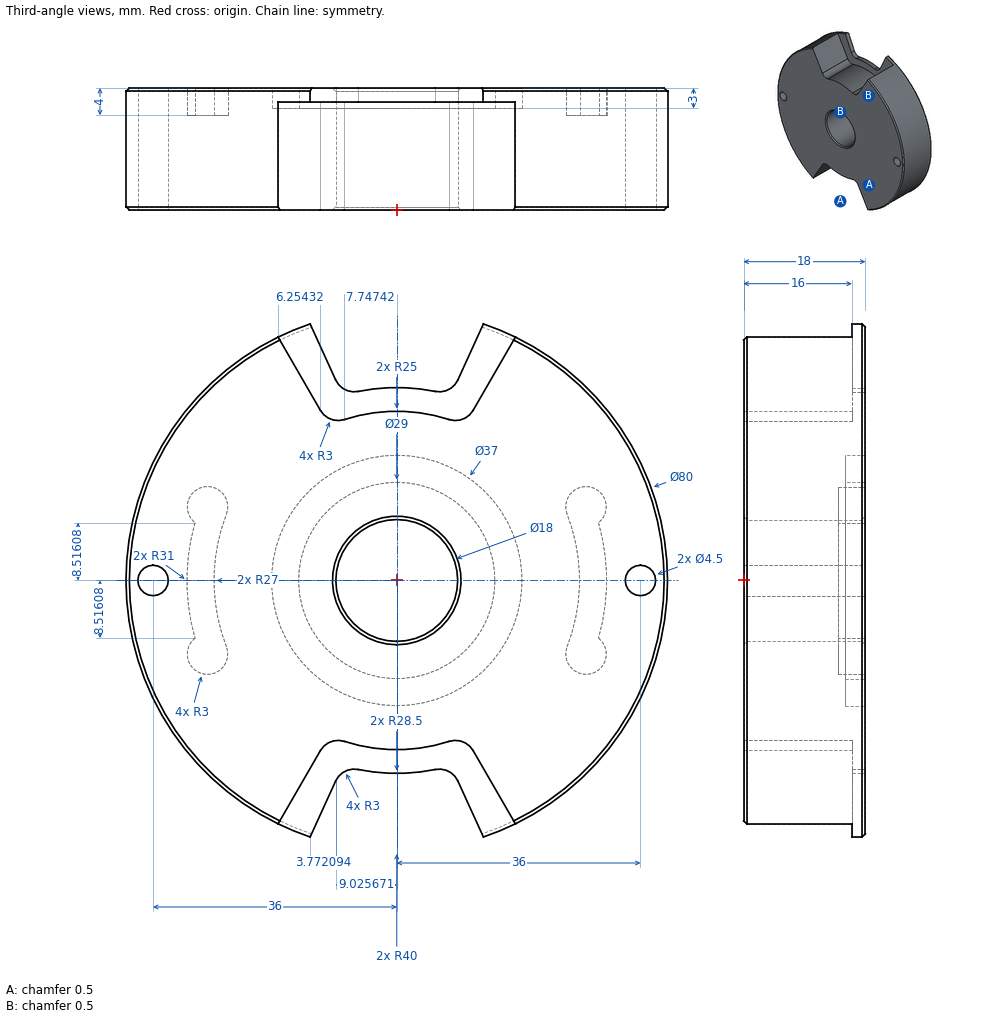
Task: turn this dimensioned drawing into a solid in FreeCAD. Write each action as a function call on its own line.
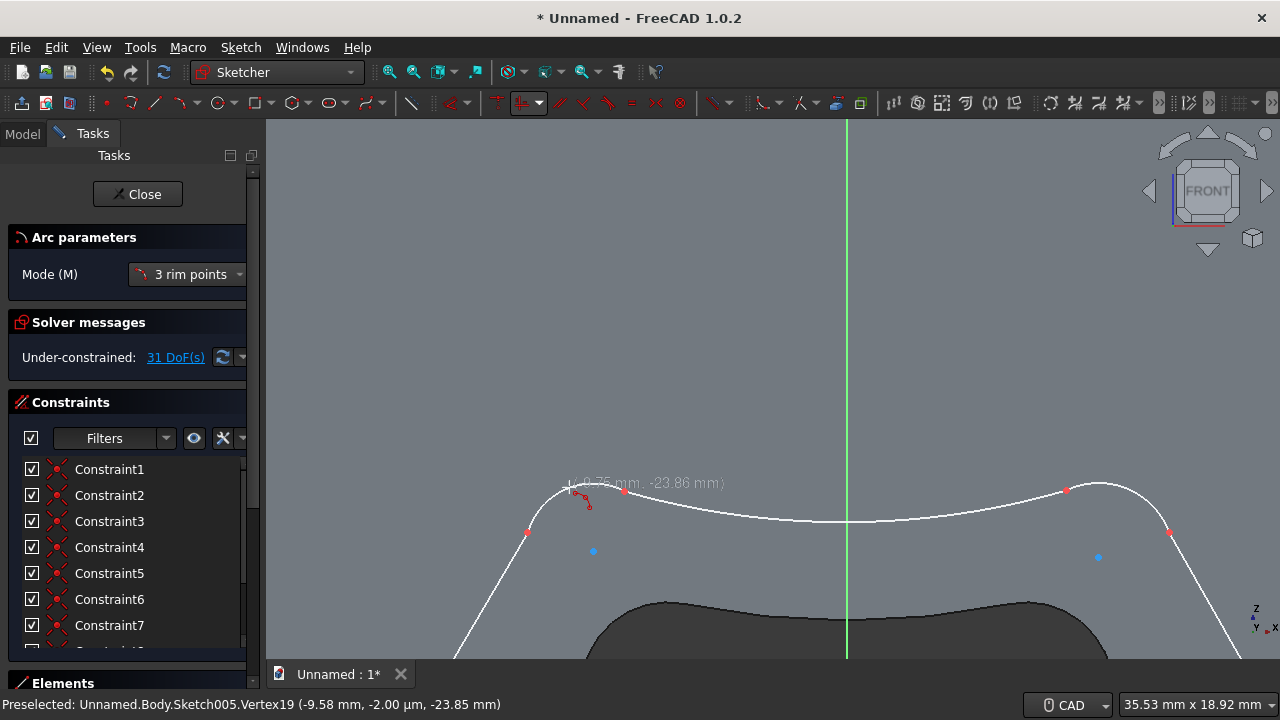
scroll(676, 504, down, 9)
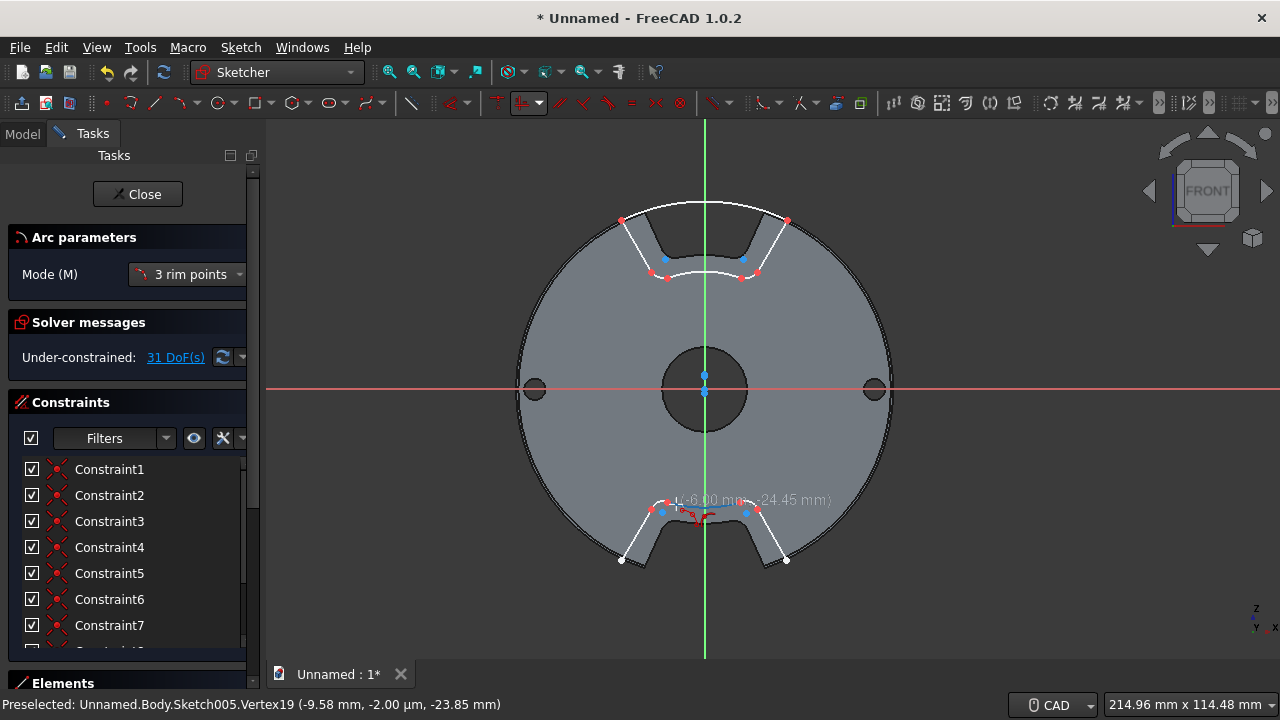
click(622, 560)
click(787, 560)
click(688, 577)
key(Escape)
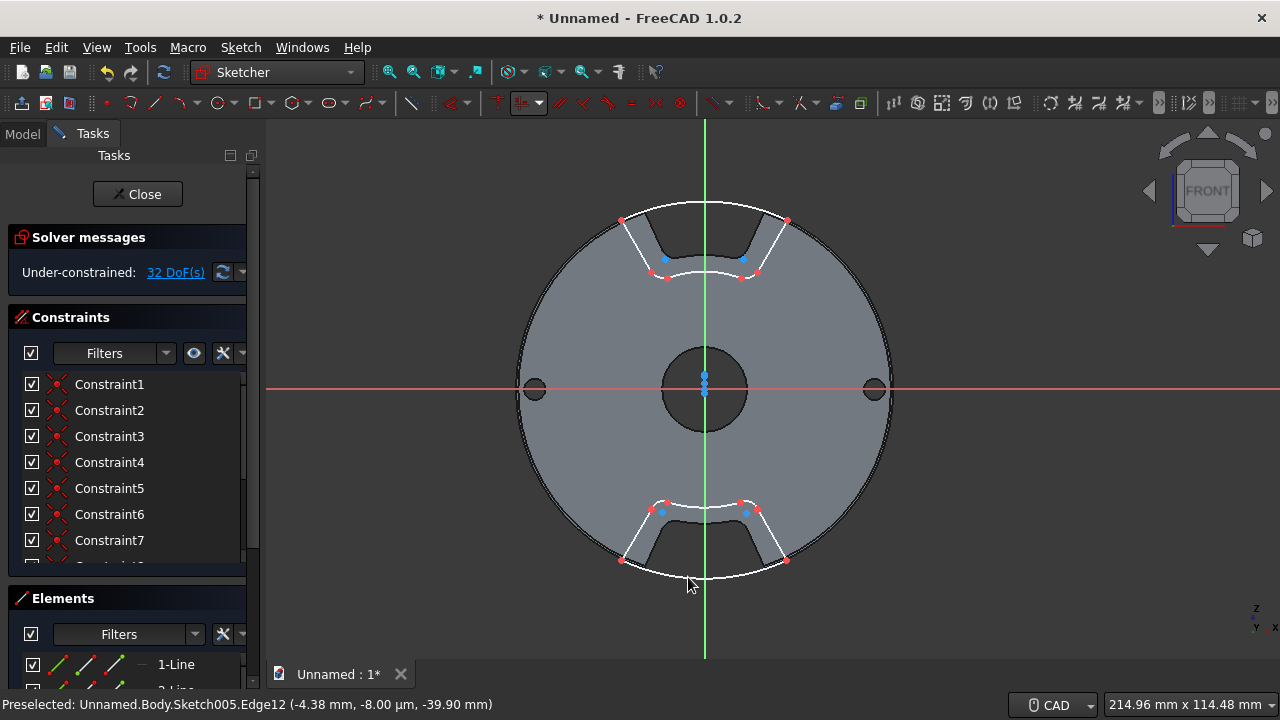
click(631, 236)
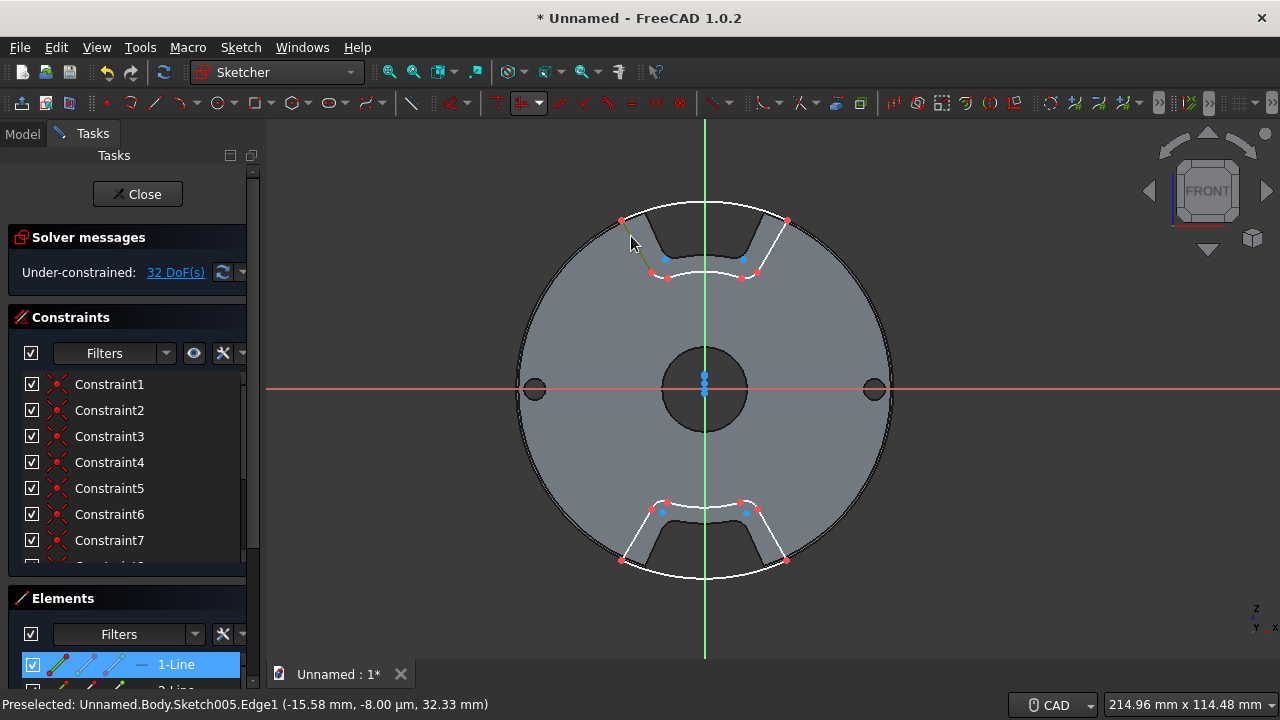
scroll(659, 277, up, 3)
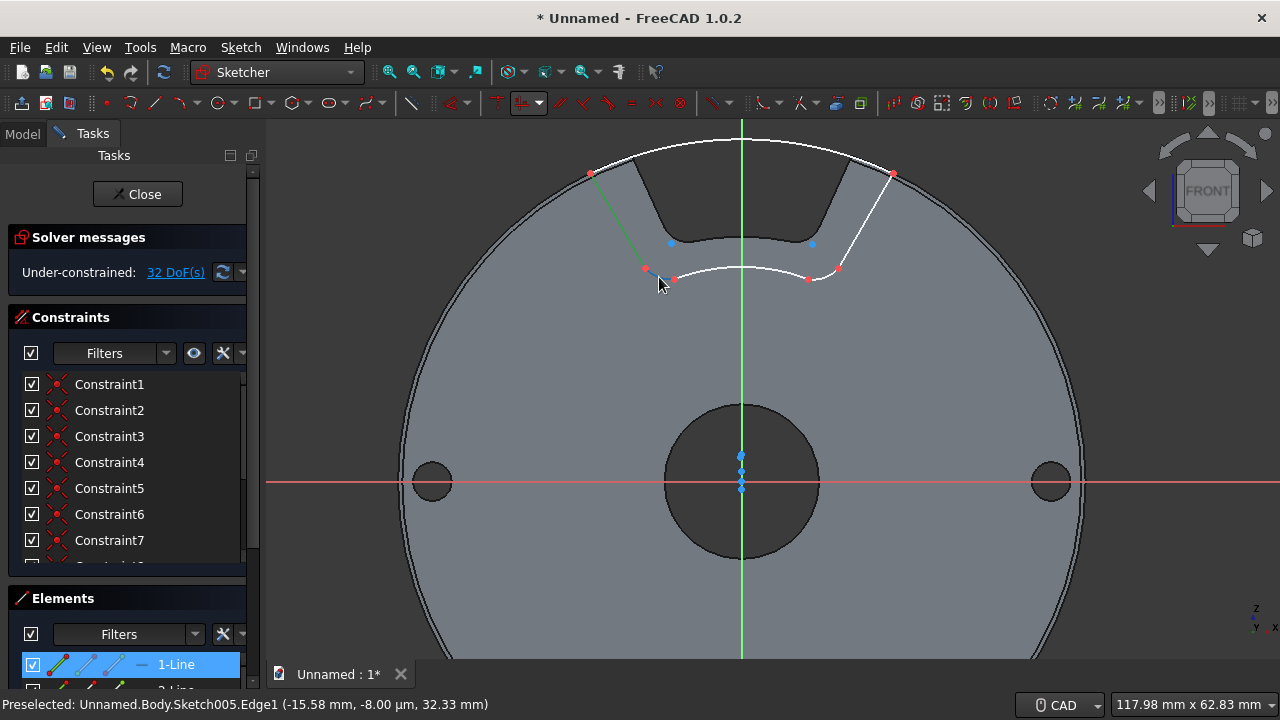
click(659, 277)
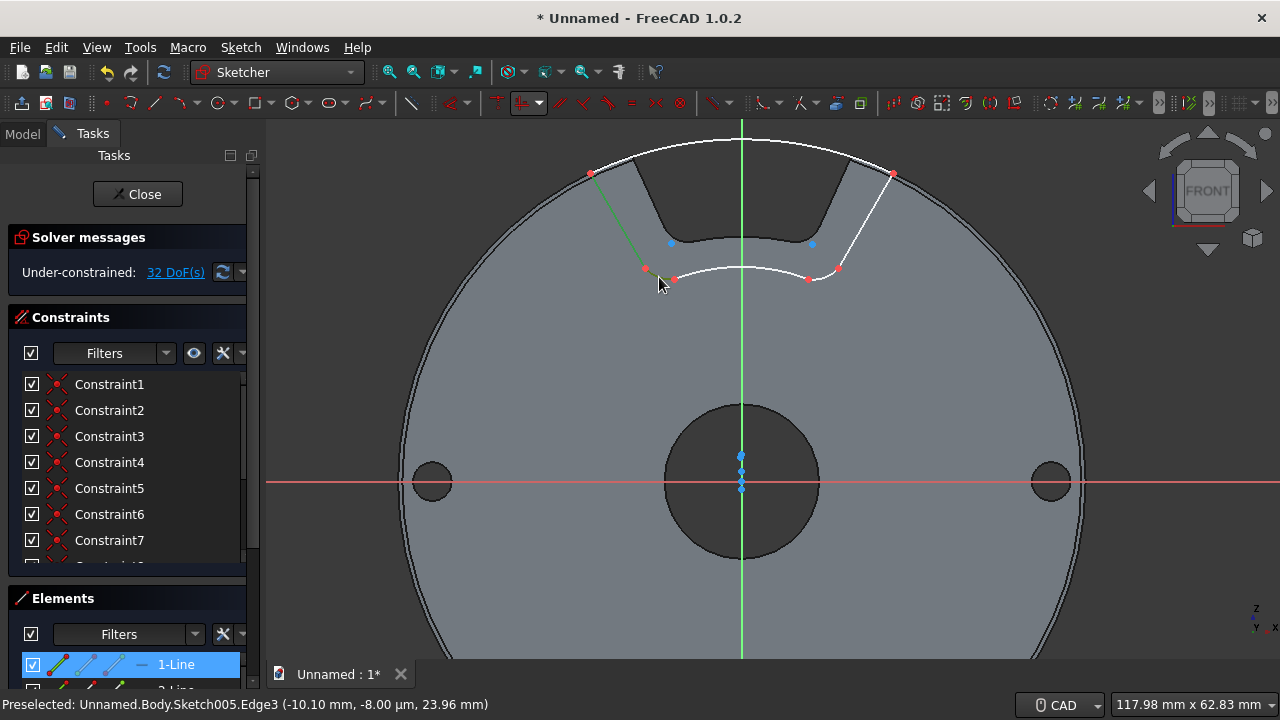
click(608, 104)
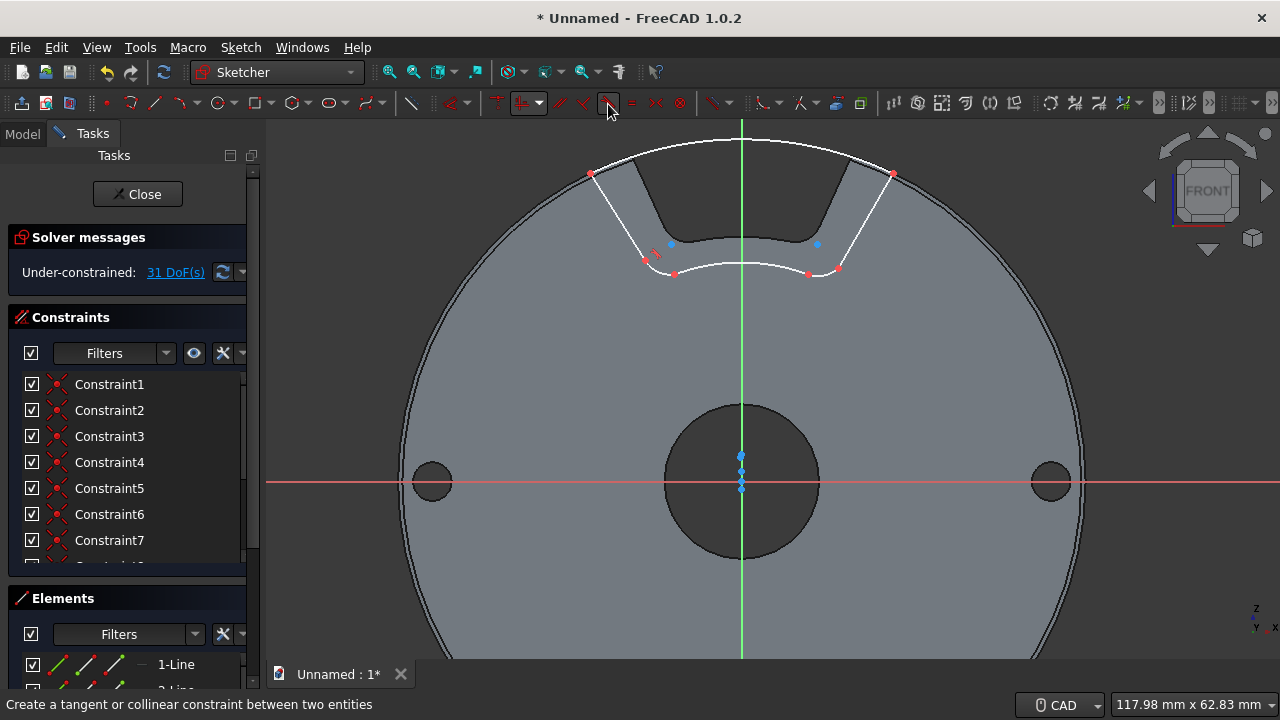
click(855, 240)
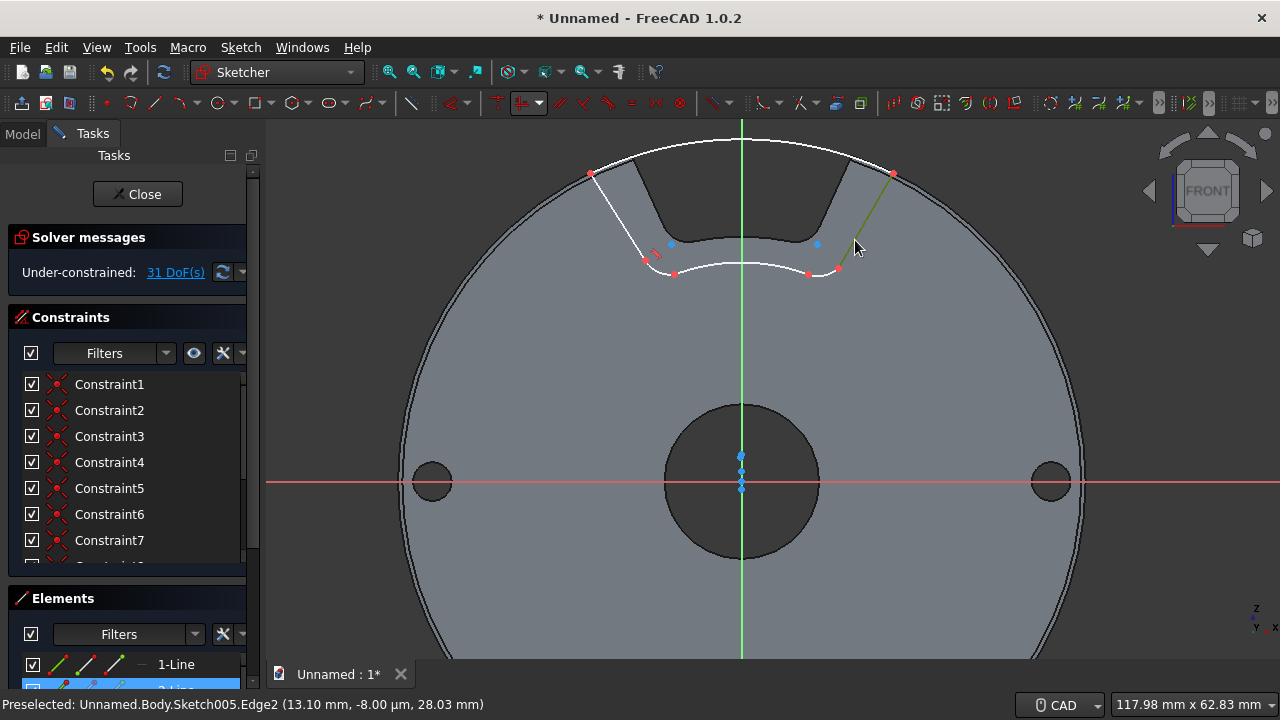
scroll(818, 276, up, 2)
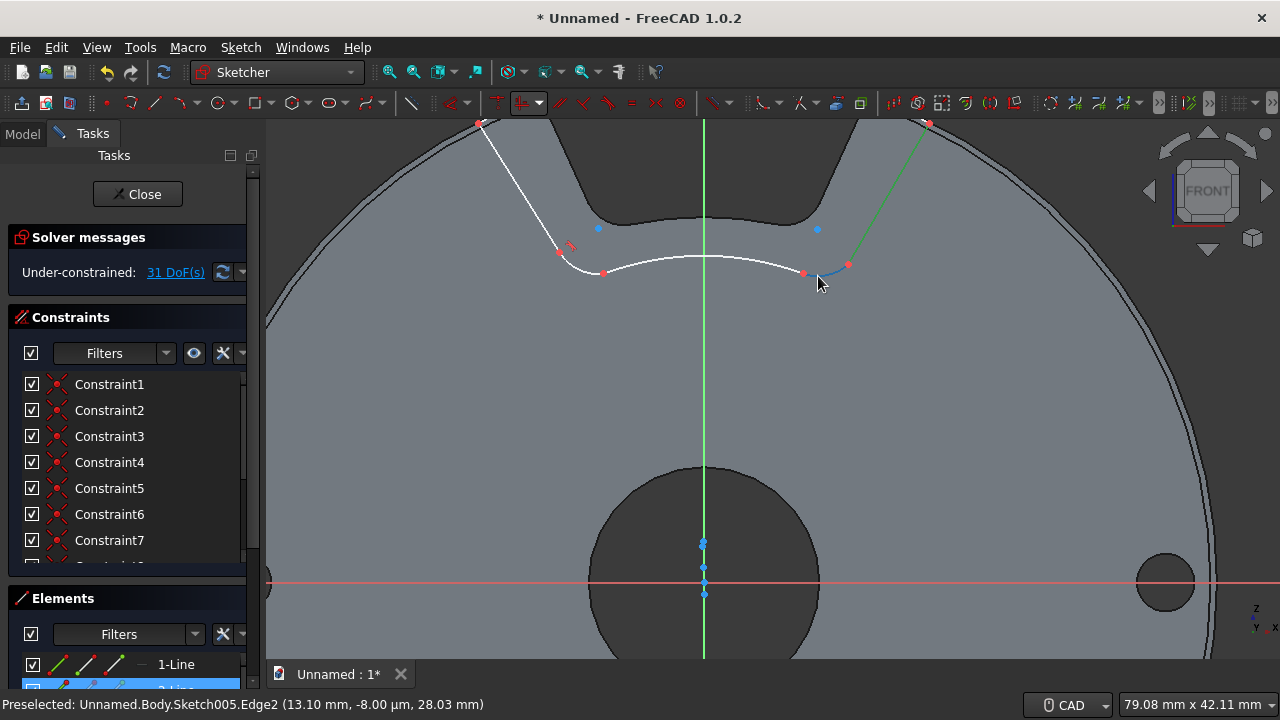
click(817, 276)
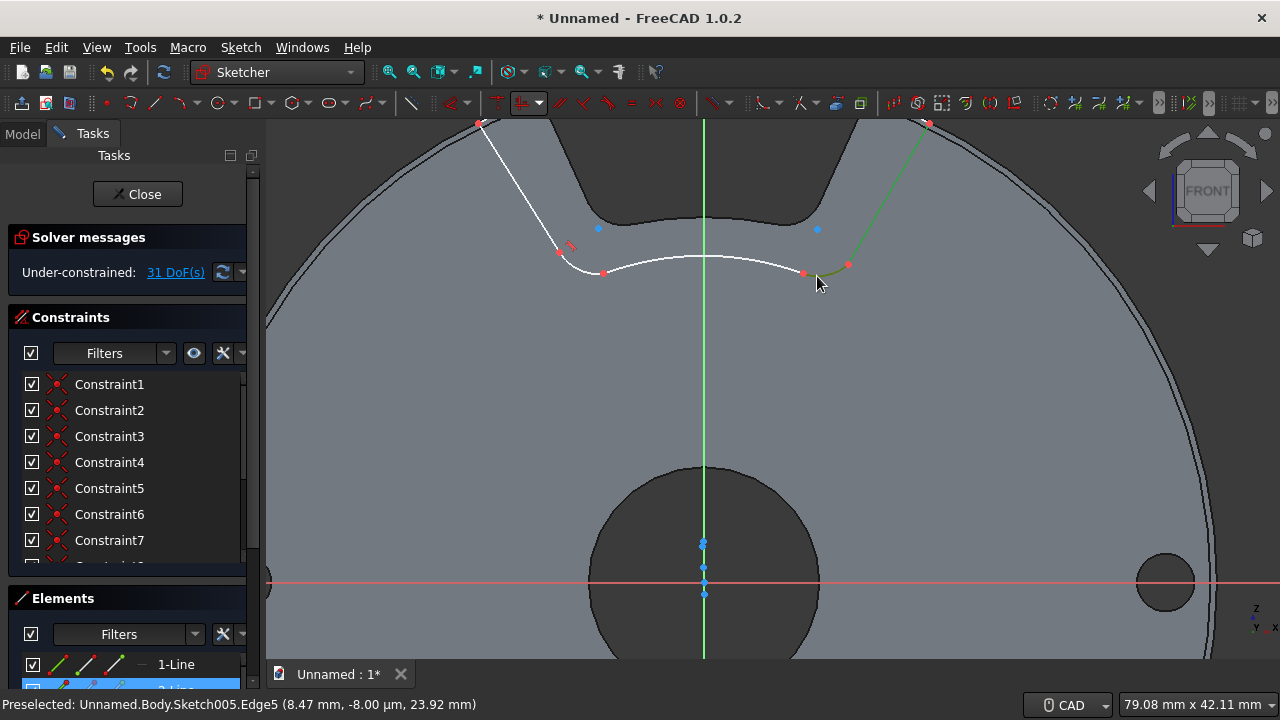
click(608, 104)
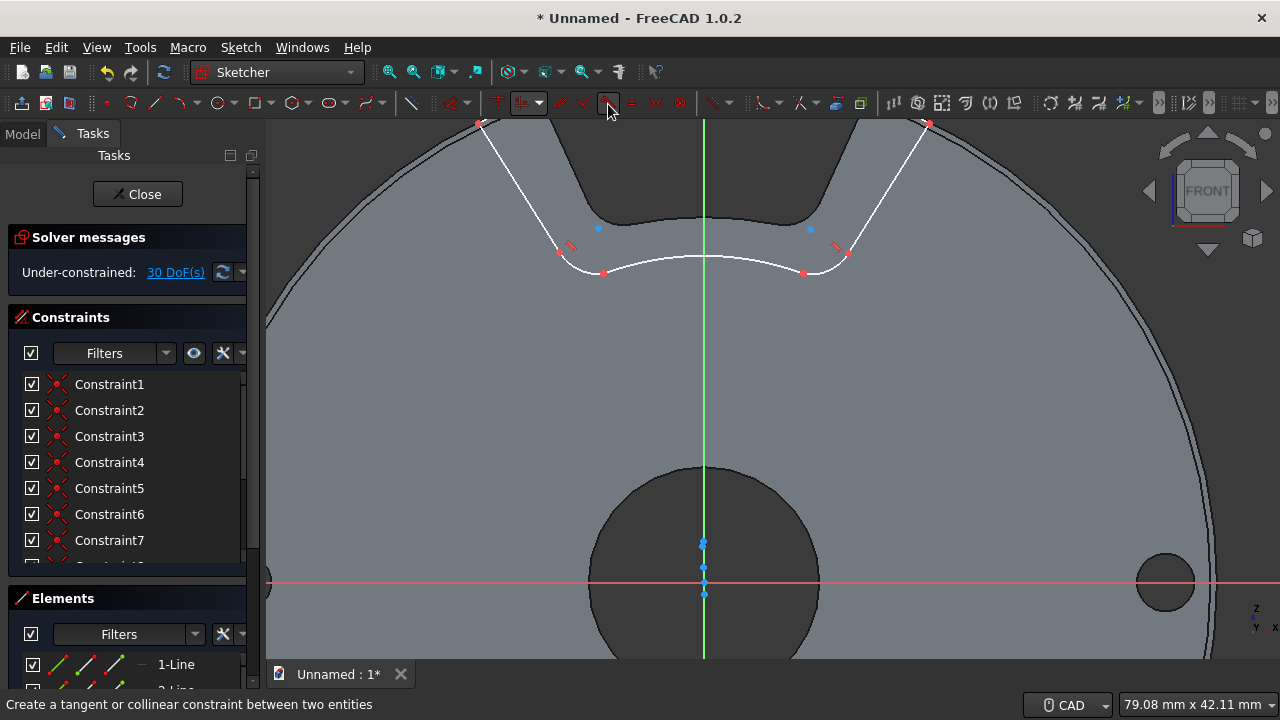
click(570, 264)